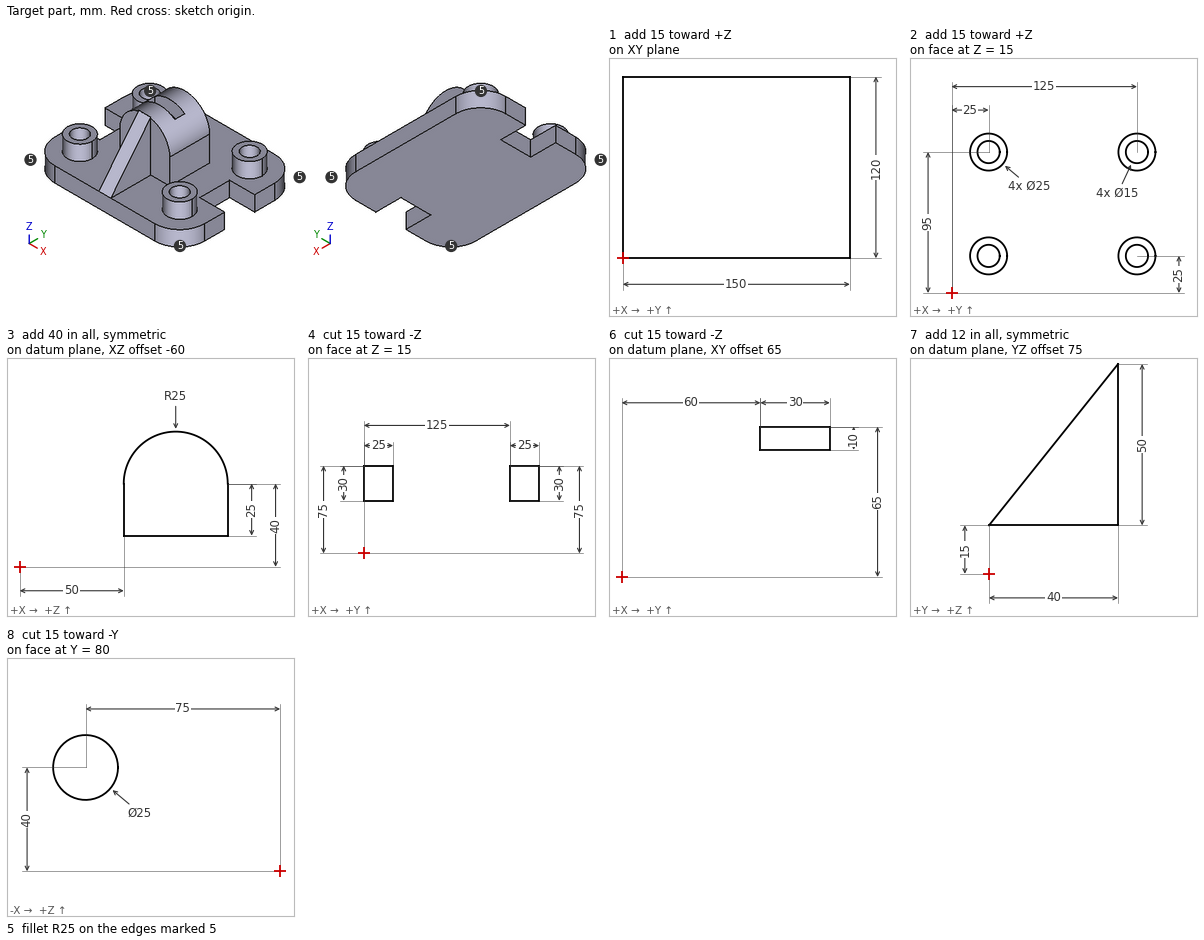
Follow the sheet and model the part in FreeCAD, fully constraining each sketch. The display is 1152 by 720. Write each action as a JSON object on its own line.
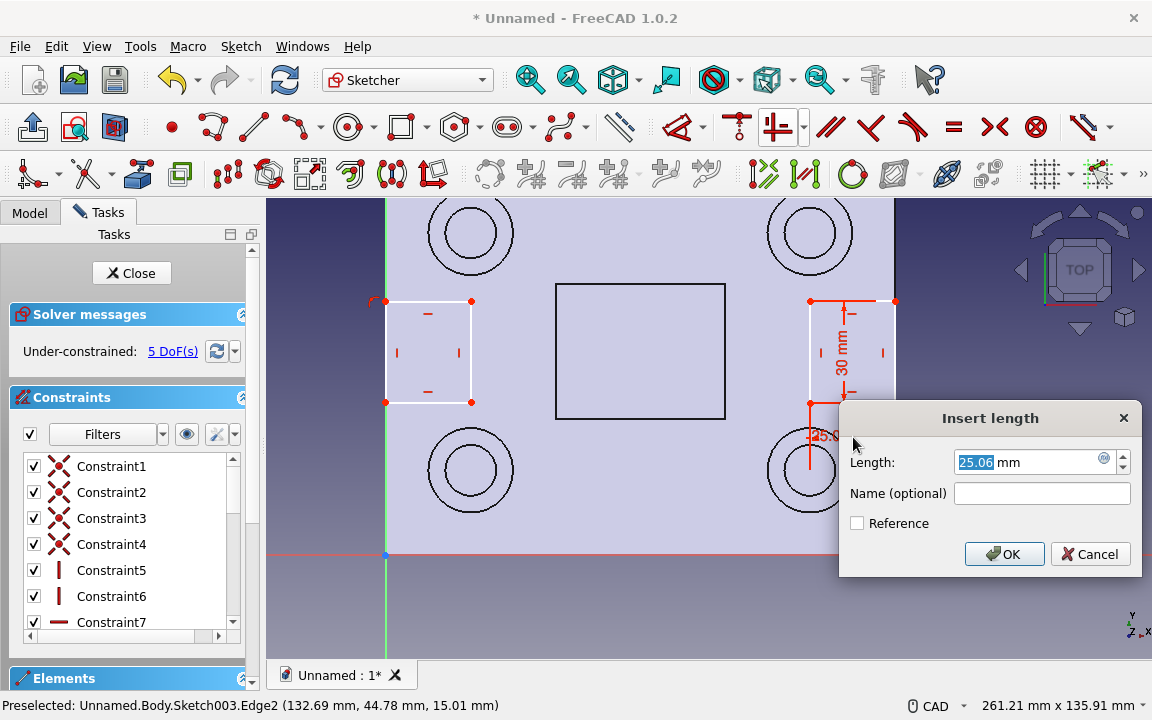
{"action": "type", "text": "25"}
{"action": "key", "text": "Return"}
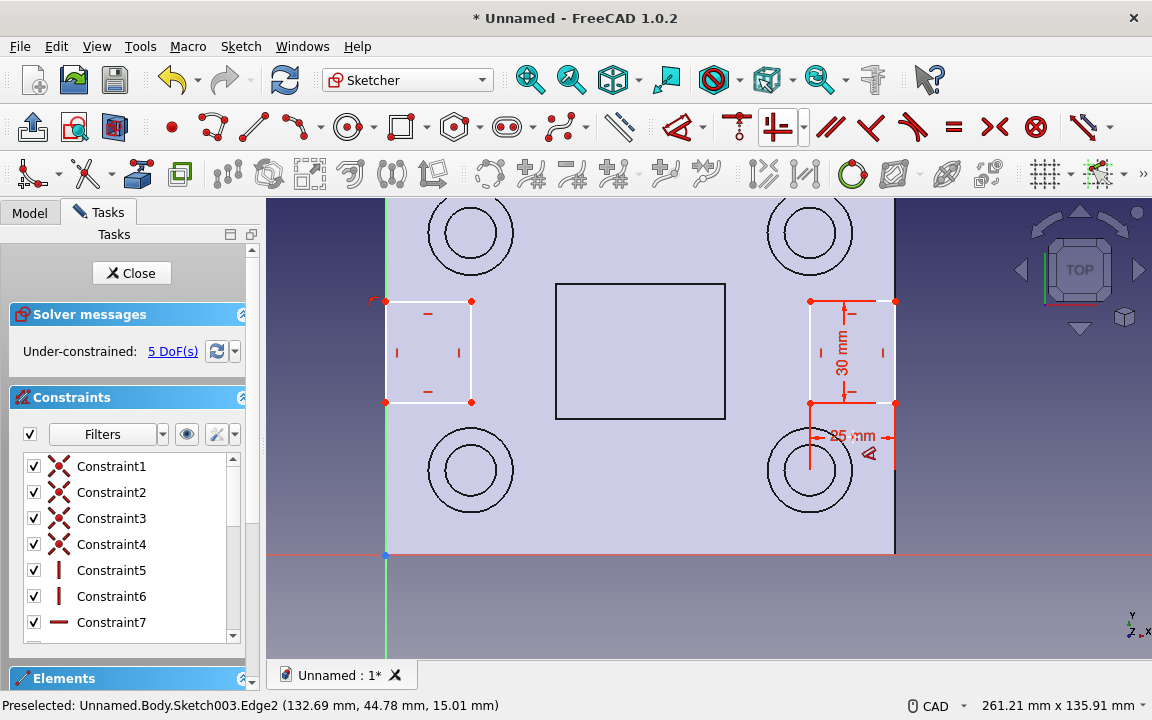
{"action": "left_click", "coordinate": [386, 332]}
{"action": "left_click", "coordinate": [352, 352]}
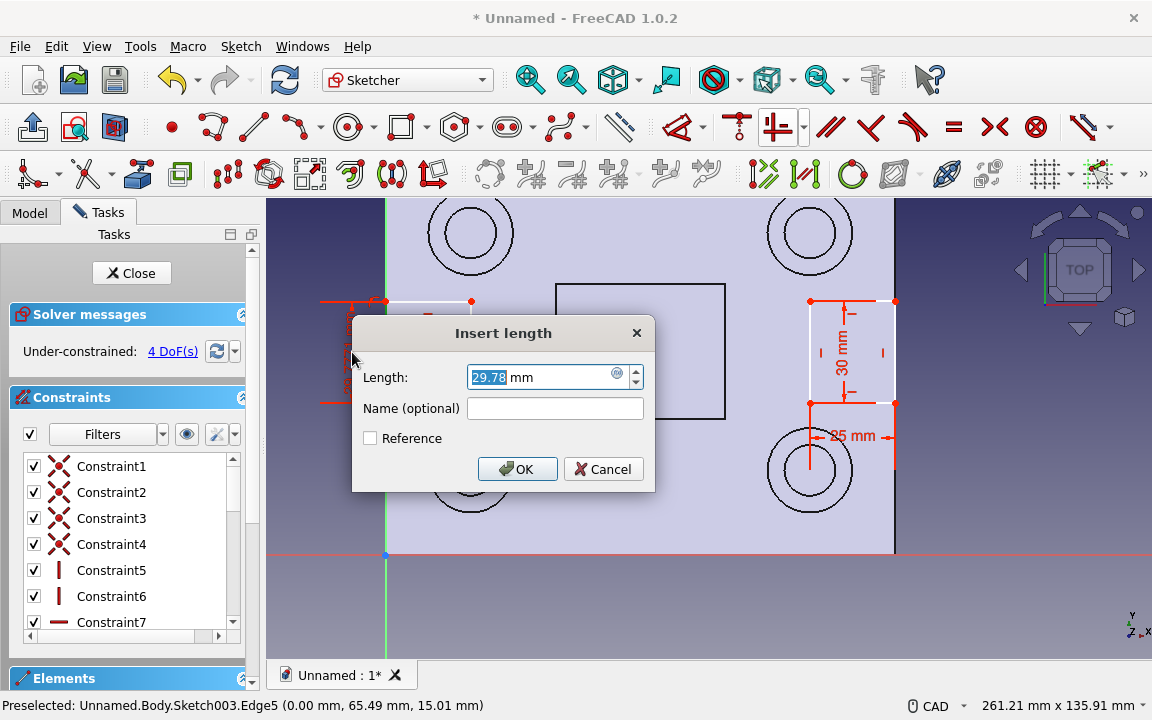
{"action": "type", "text": "30"}
{"action": "key", "text": "Return"}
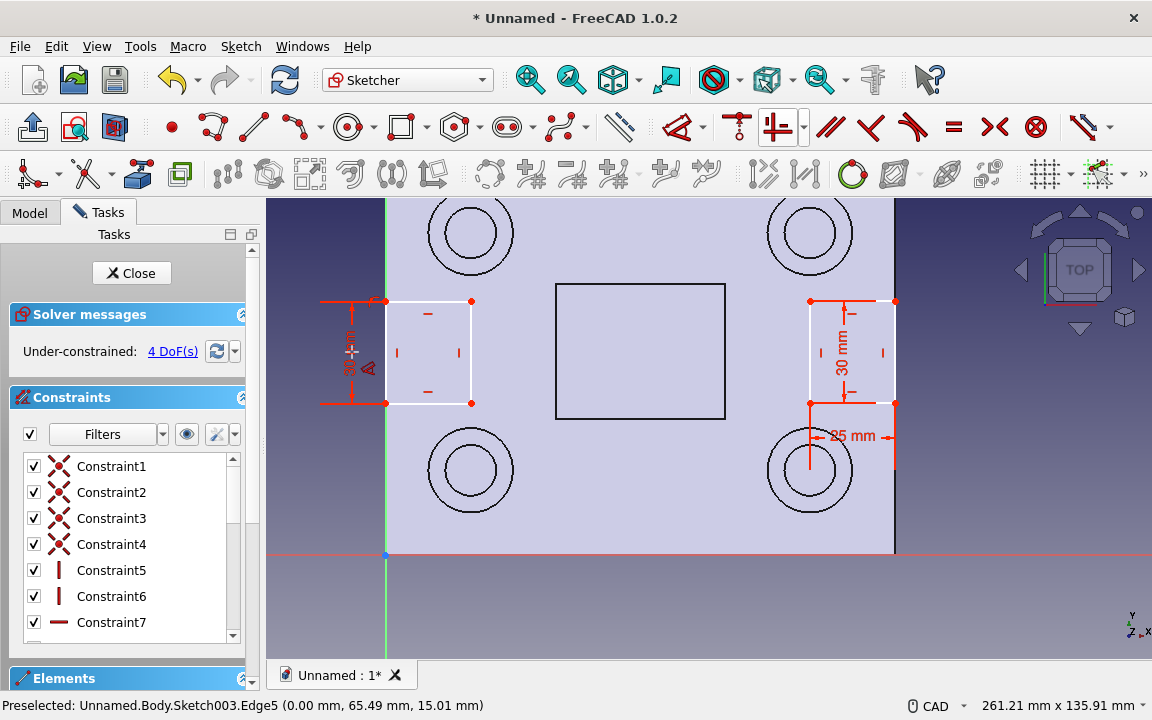
{"action": "left_click", "coordinate": [411, 404]}
{"action": "left_click", "coordinate": [428, 370]}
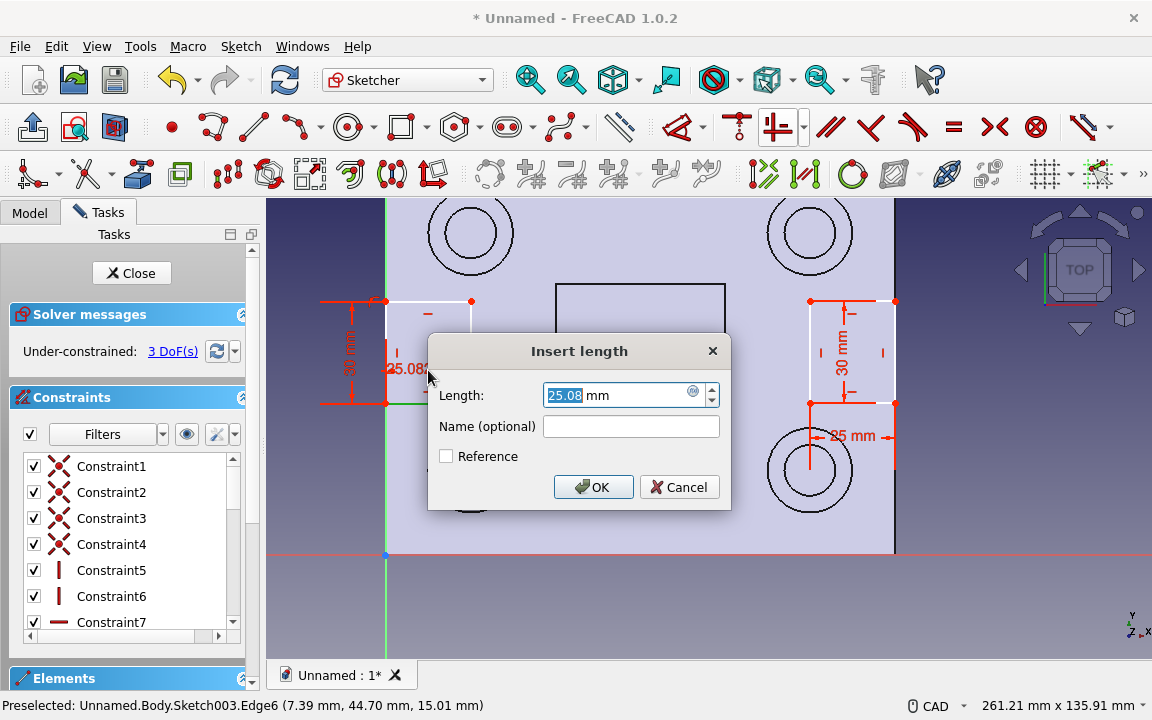
{"action": "type", "text": "25"}
{"action": "key", "text": "Return"}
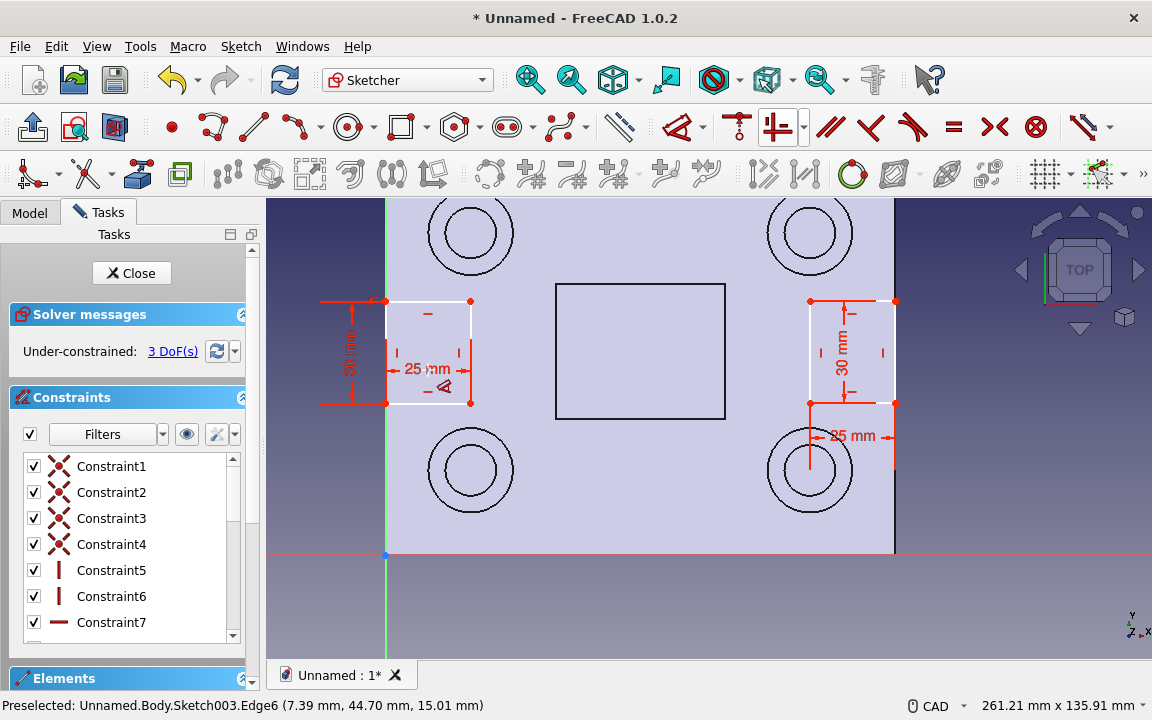
{"action": "left_click", "coordinate": [810, 301]}
{"action": "left_click", "coordinate": [352, 428]}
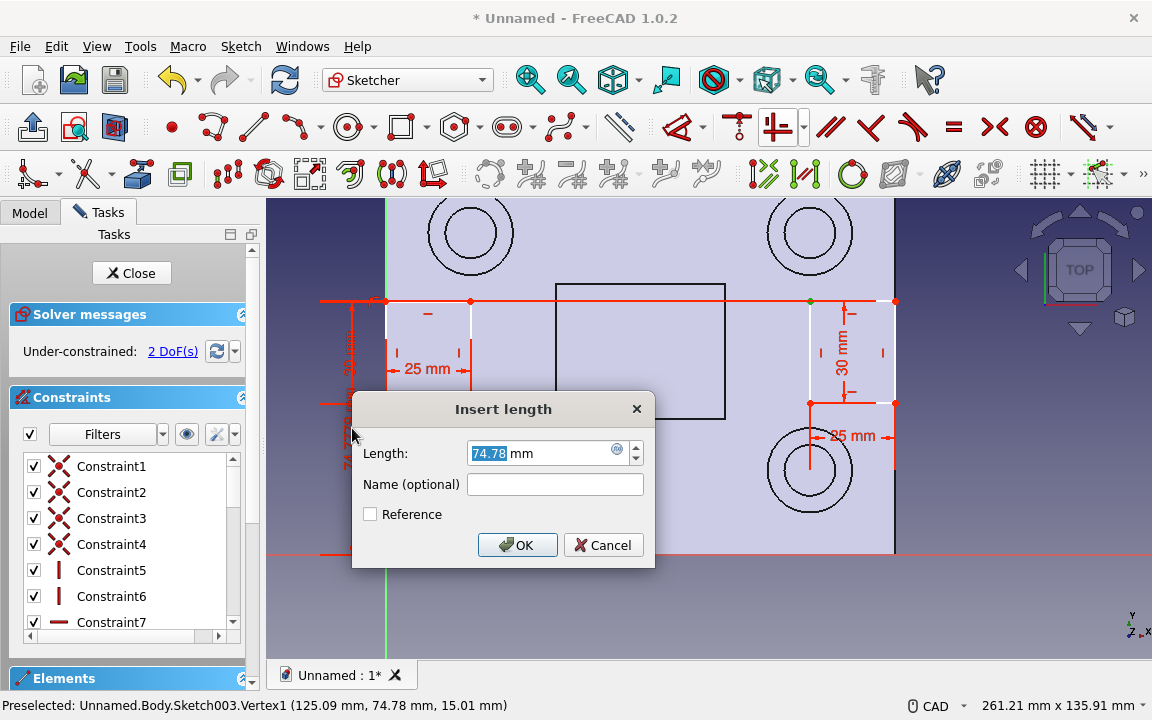
{"action": "type", "text": "75"}
{"action": "key", "text": "Return"}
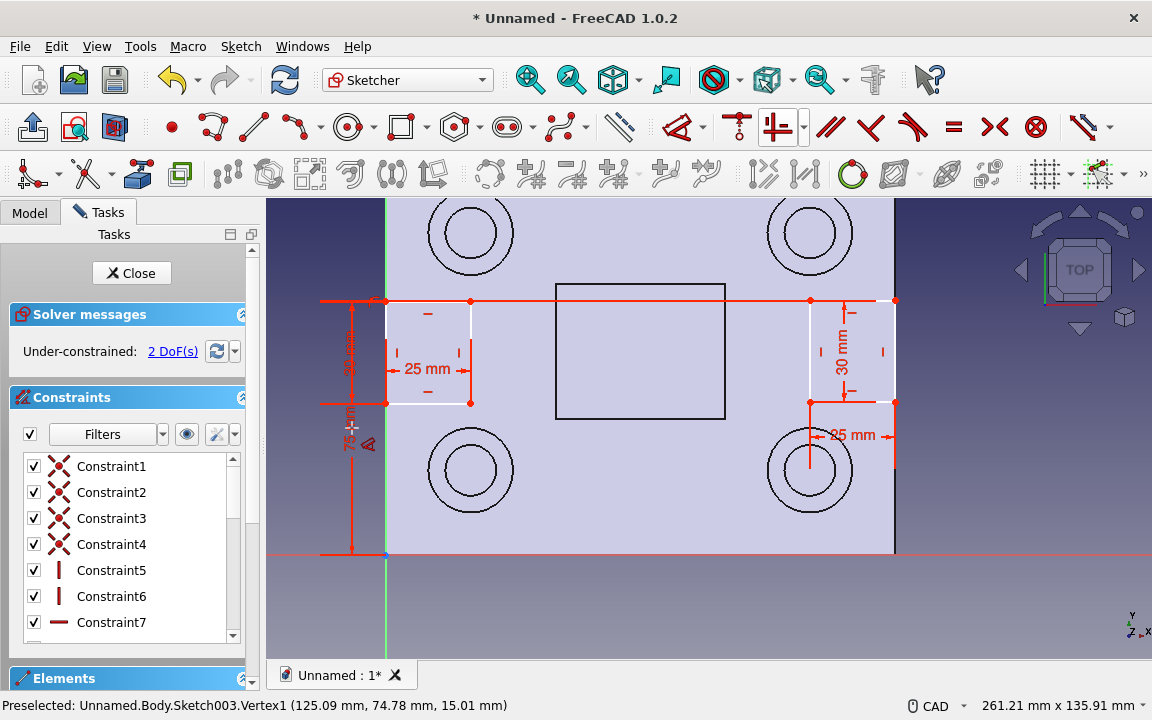
{"action": "left_click", "coordinate": [386, 302]}
{"action": "left_click", "coordinate": [352, 487]}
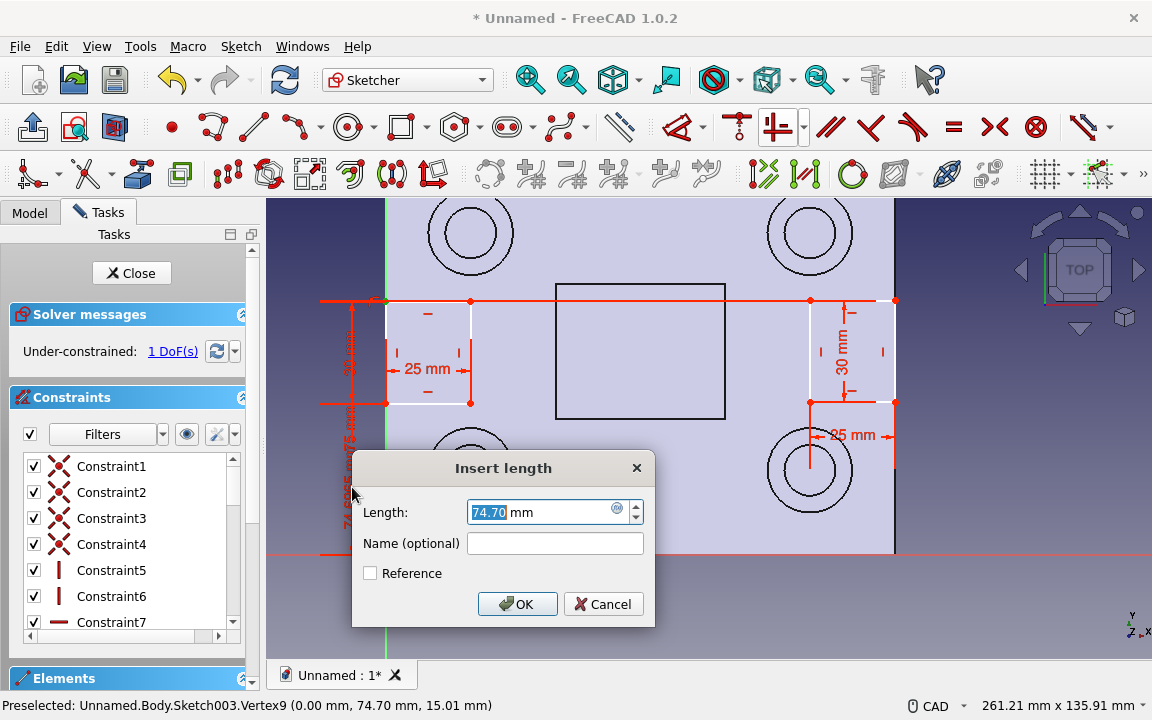
{"action": "type", "text": "75"}
{"action": "key", "text": "Return"}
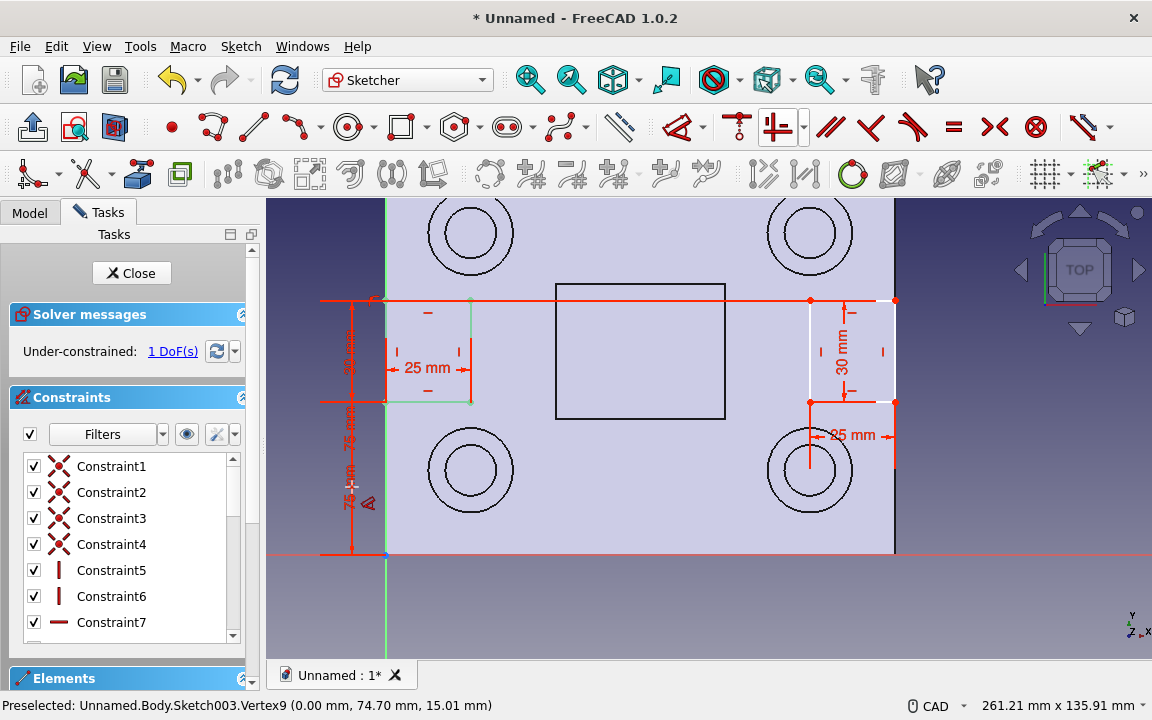
{"action": "left_click", "coordinate": [810, 301]}
{"action": "left_click", "coordinate": [598, 589]}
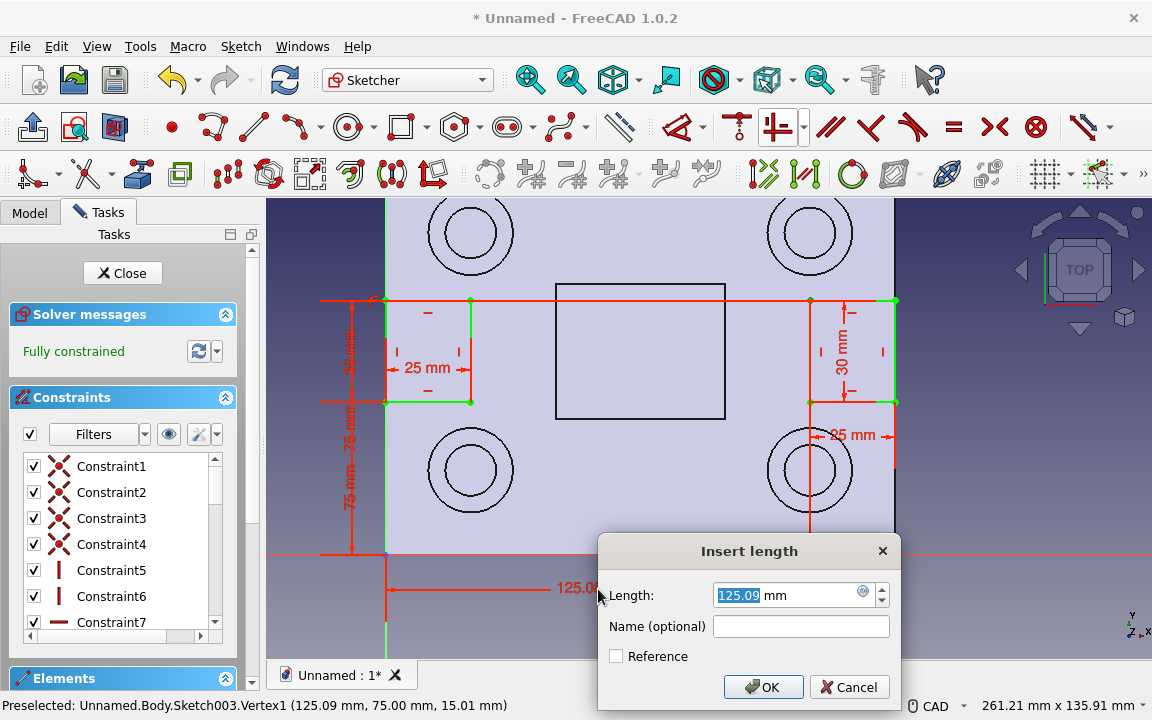
{"action": "type", "text": "125"}
{"action": "key", "text": "Return"}
{"action": "key", "text": "Escape"}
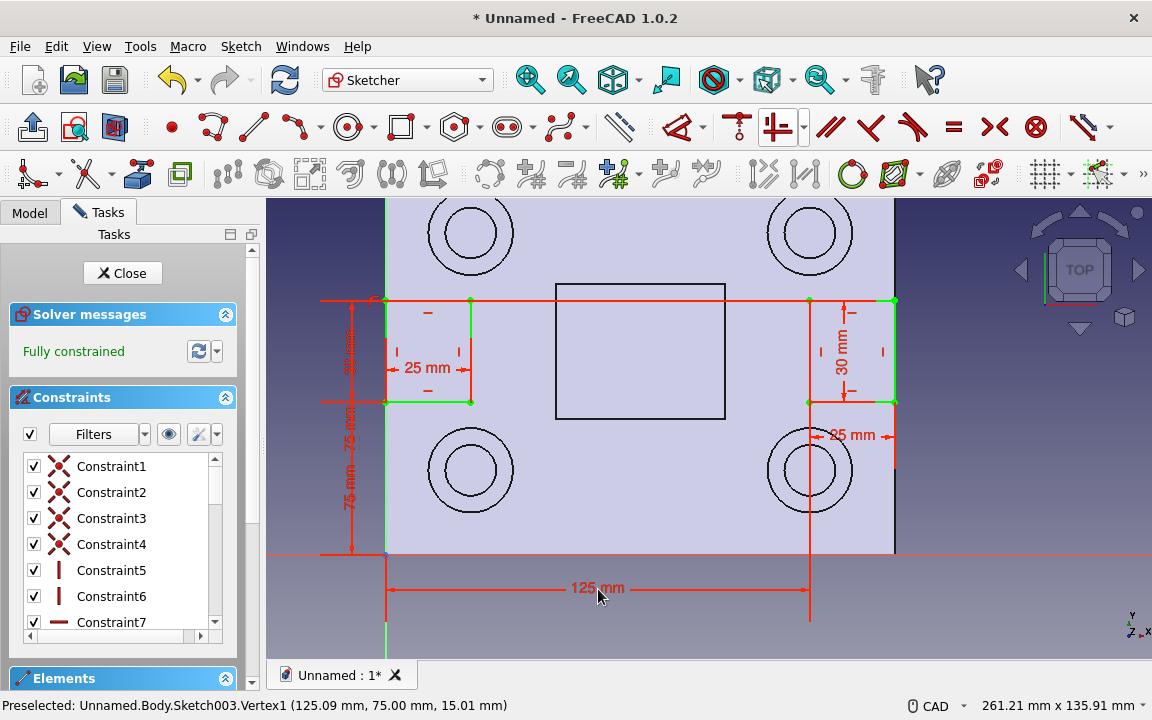
{"action": "left_click", "coordinate": [123, 273]}